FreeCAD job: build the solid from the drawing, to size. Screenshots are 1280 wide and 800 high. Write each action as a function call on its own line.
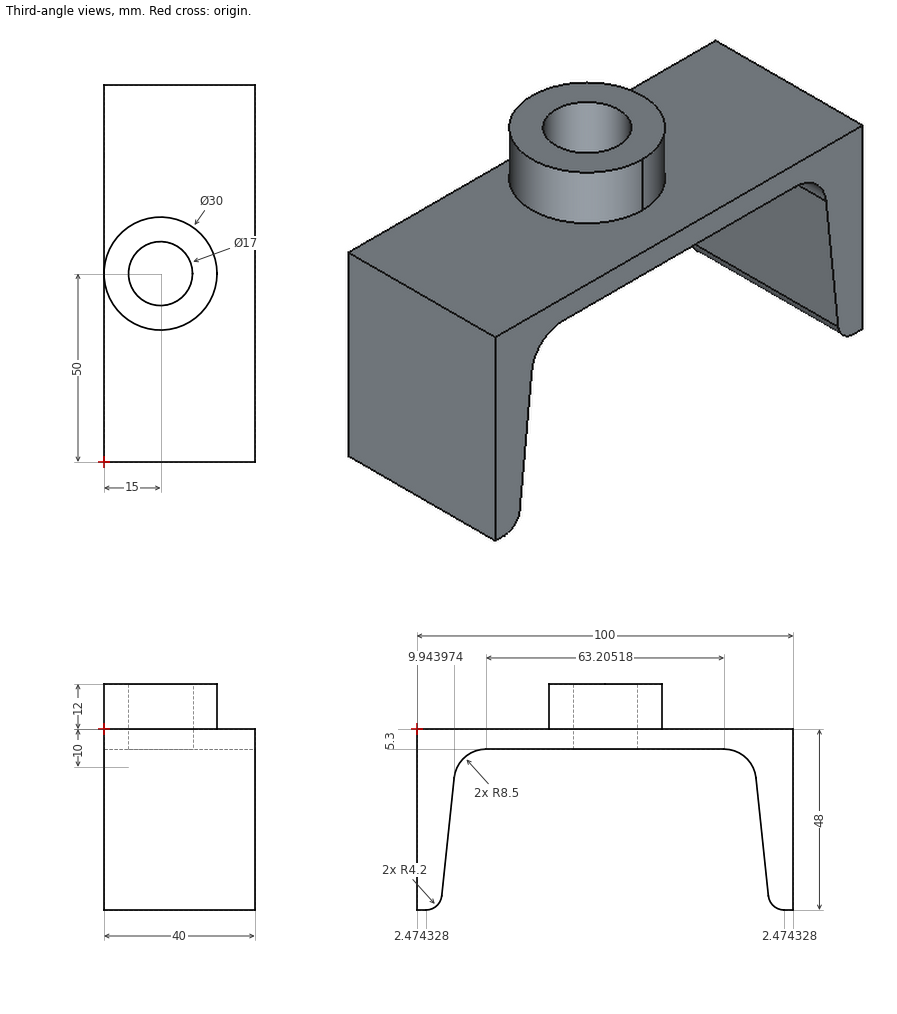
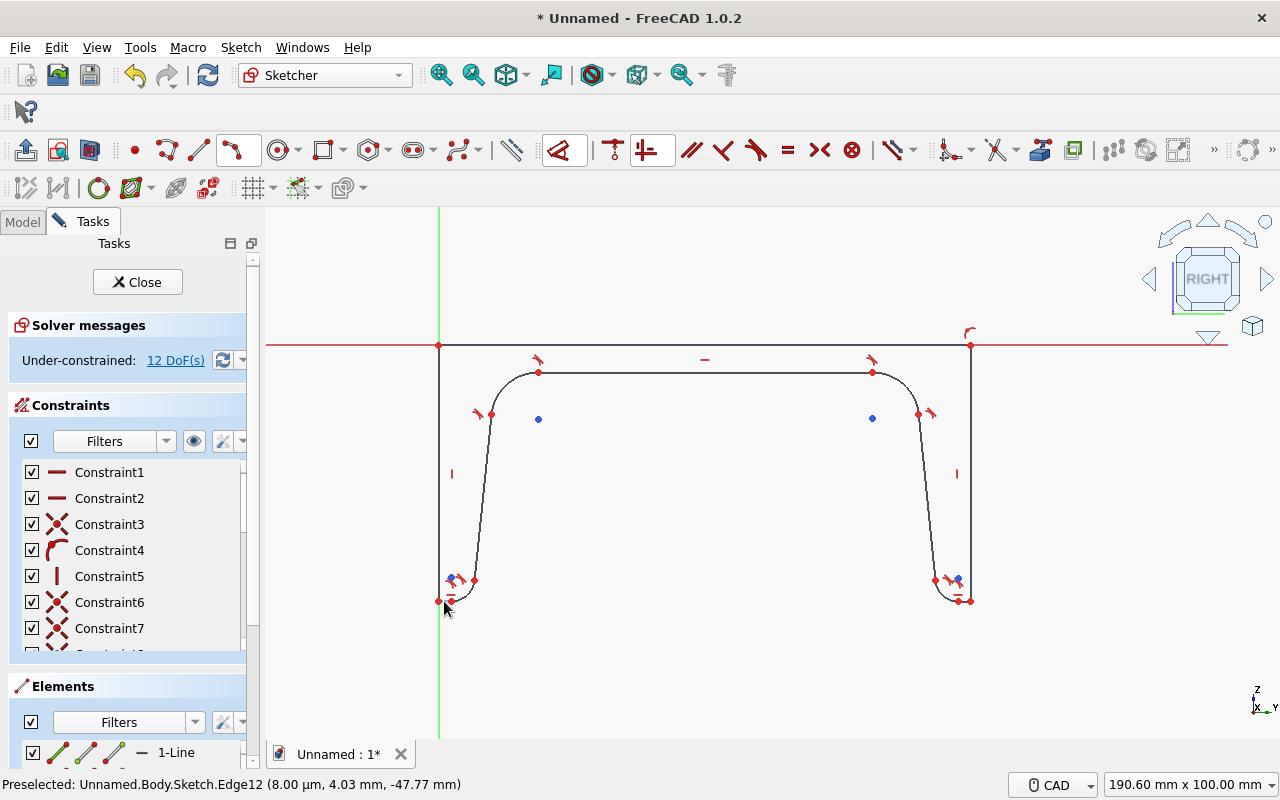
click(518, 377)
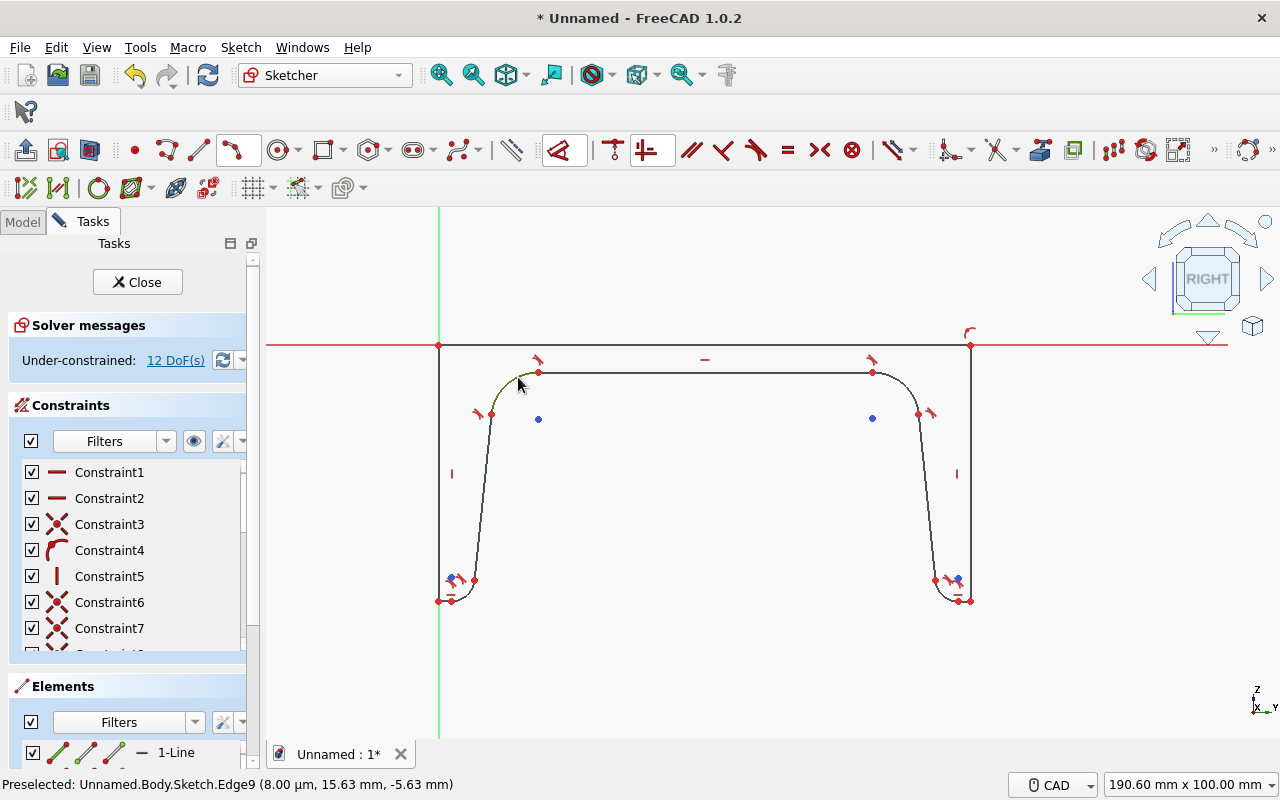
click(912, 395)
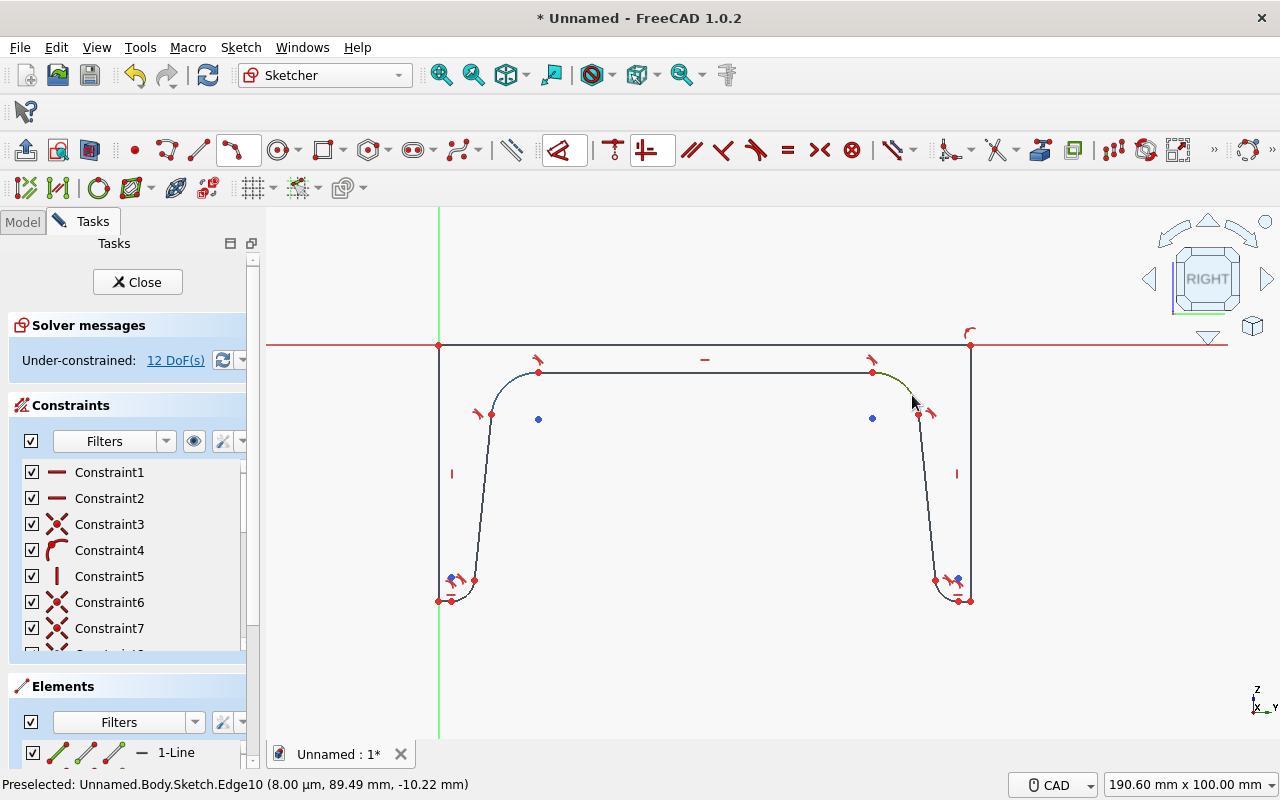
click(788, 150)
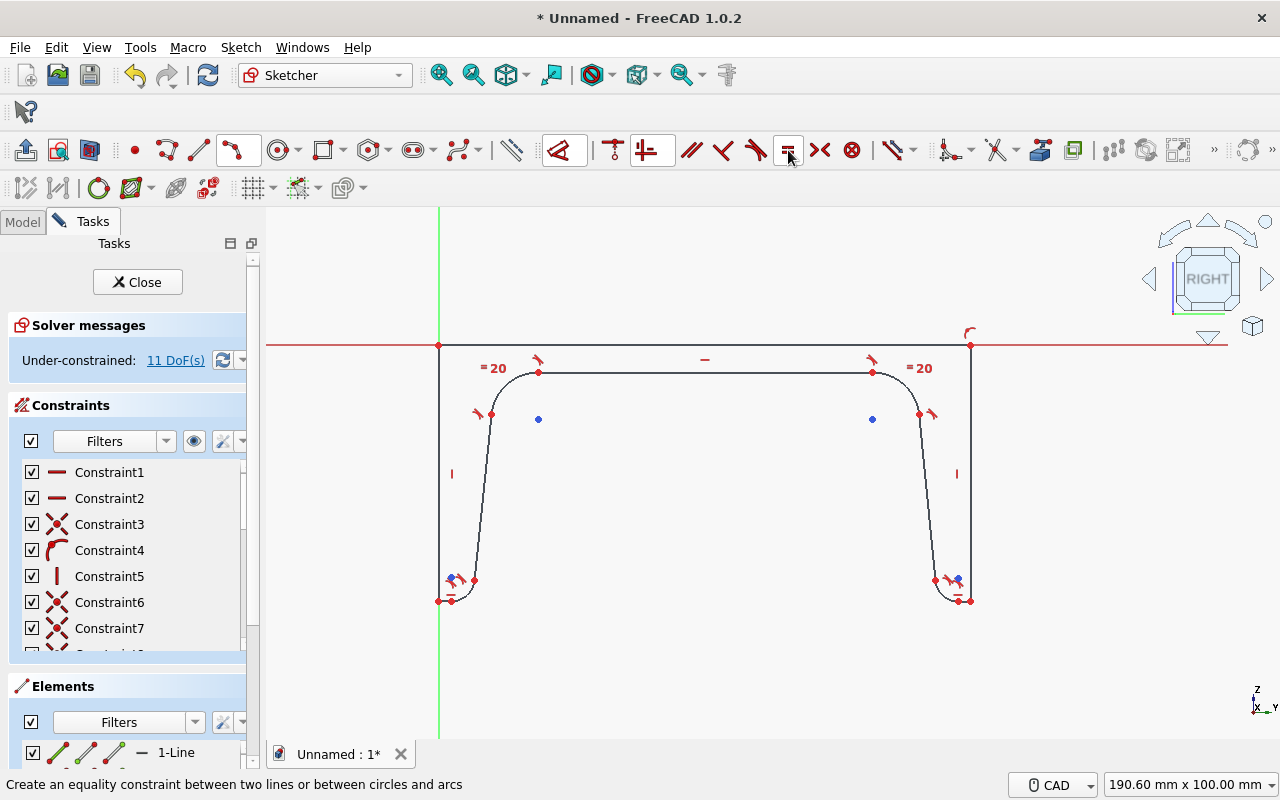
scroll(939, 590, up, 2)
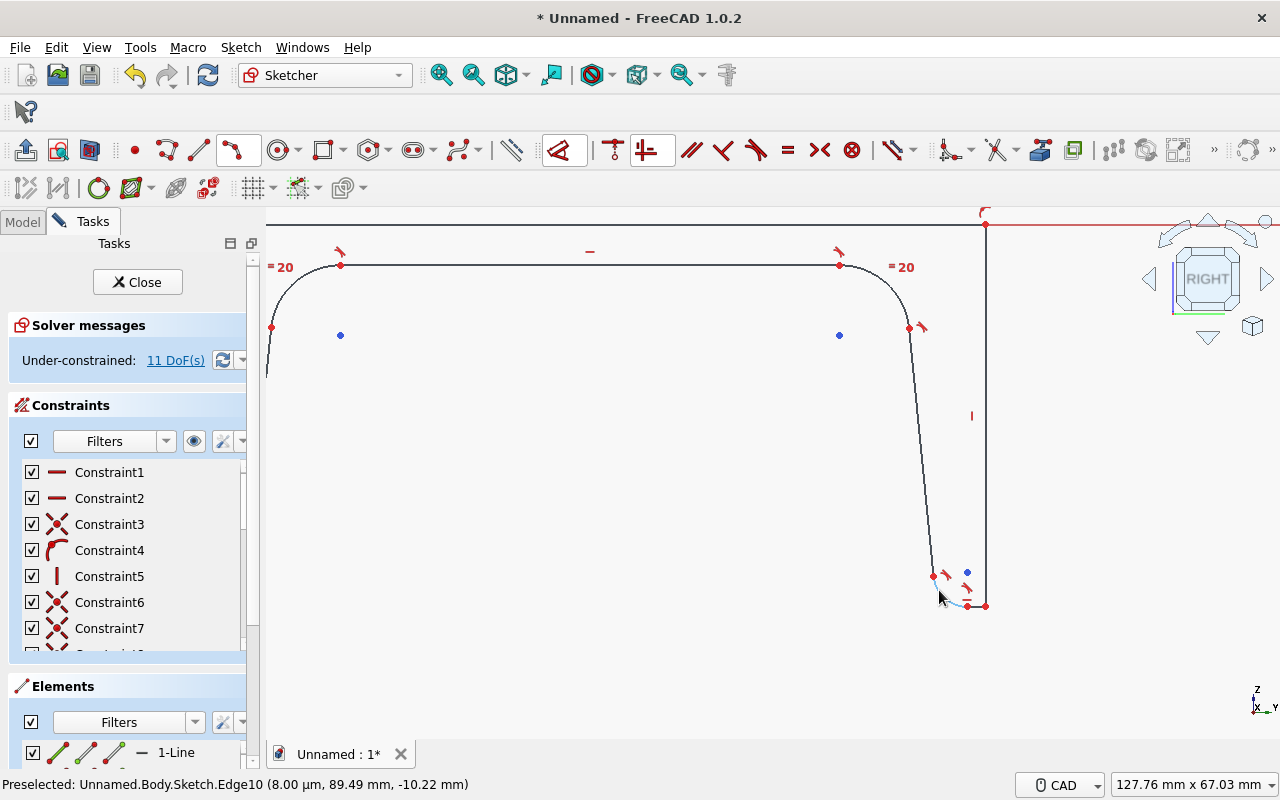
click(938, 590)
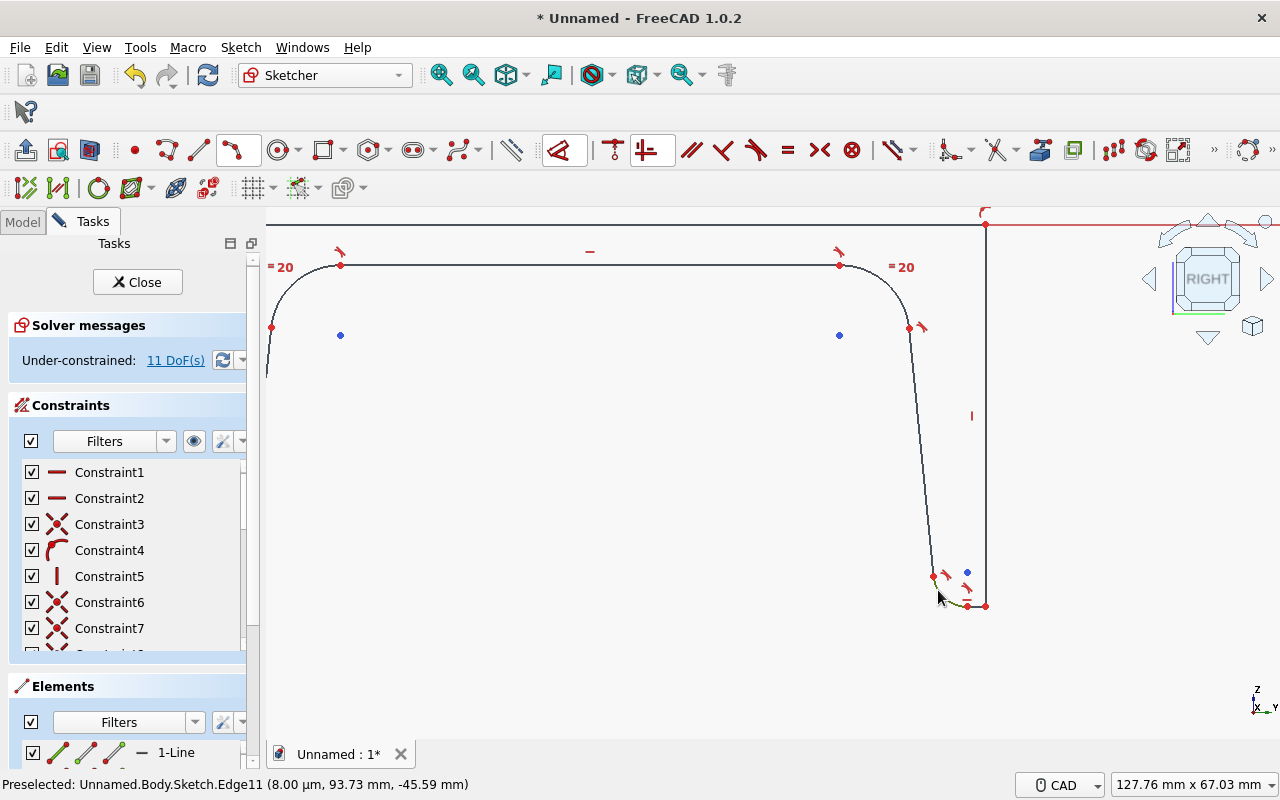
scroll(939, 590, down, 2)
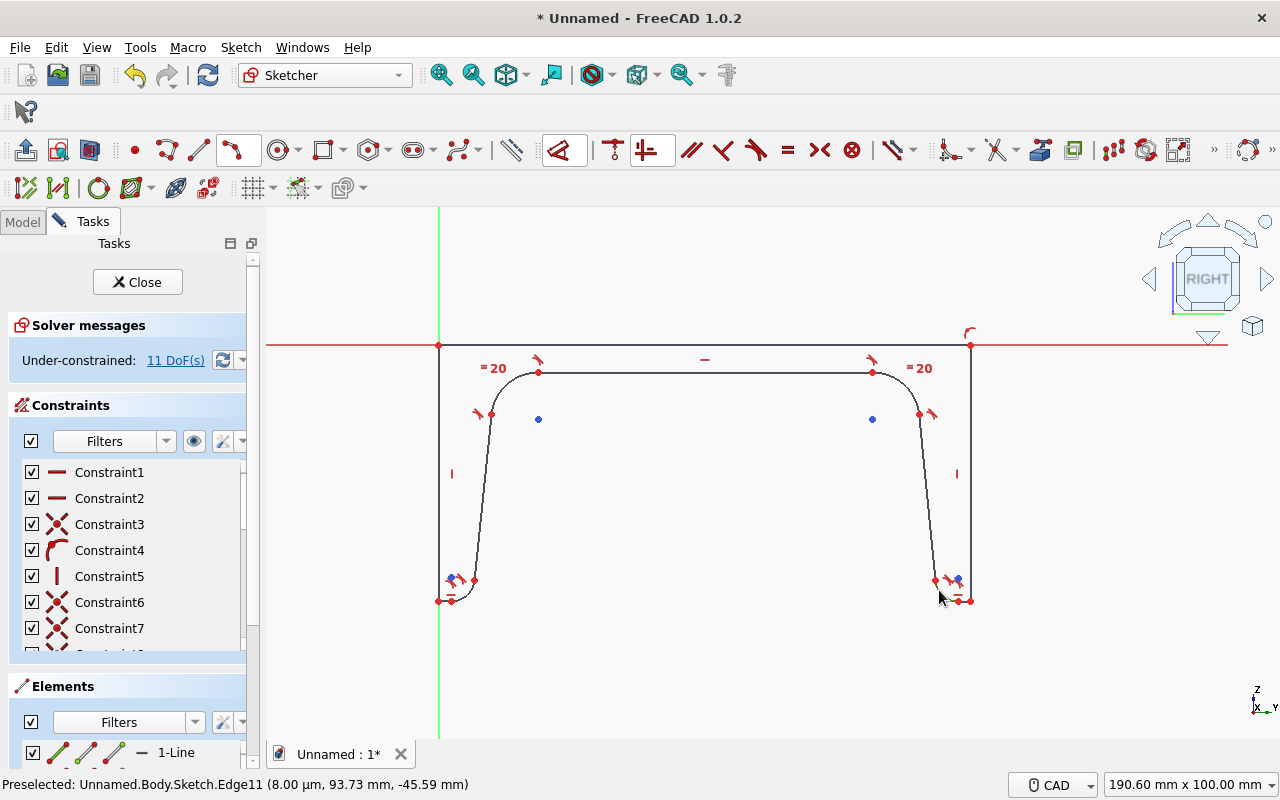
scroll(461, 599, up, 2)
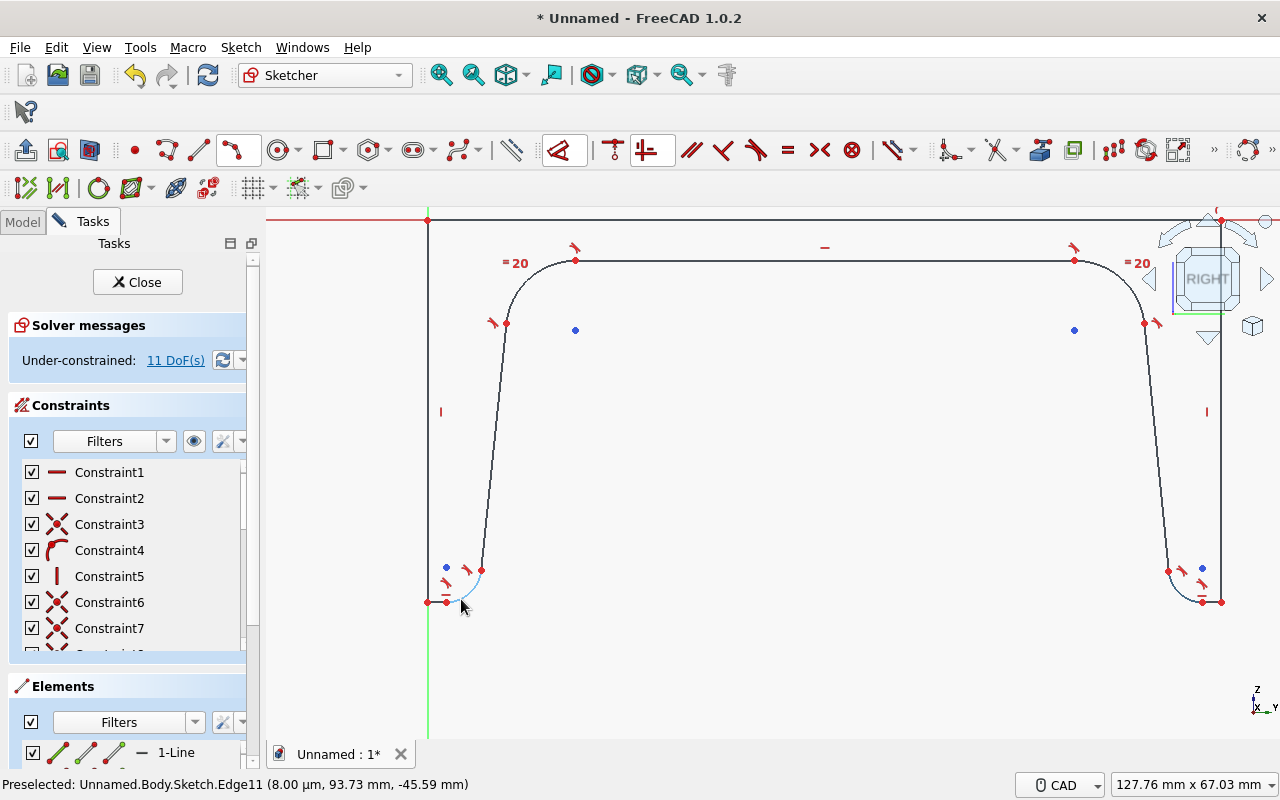
click(461, 599)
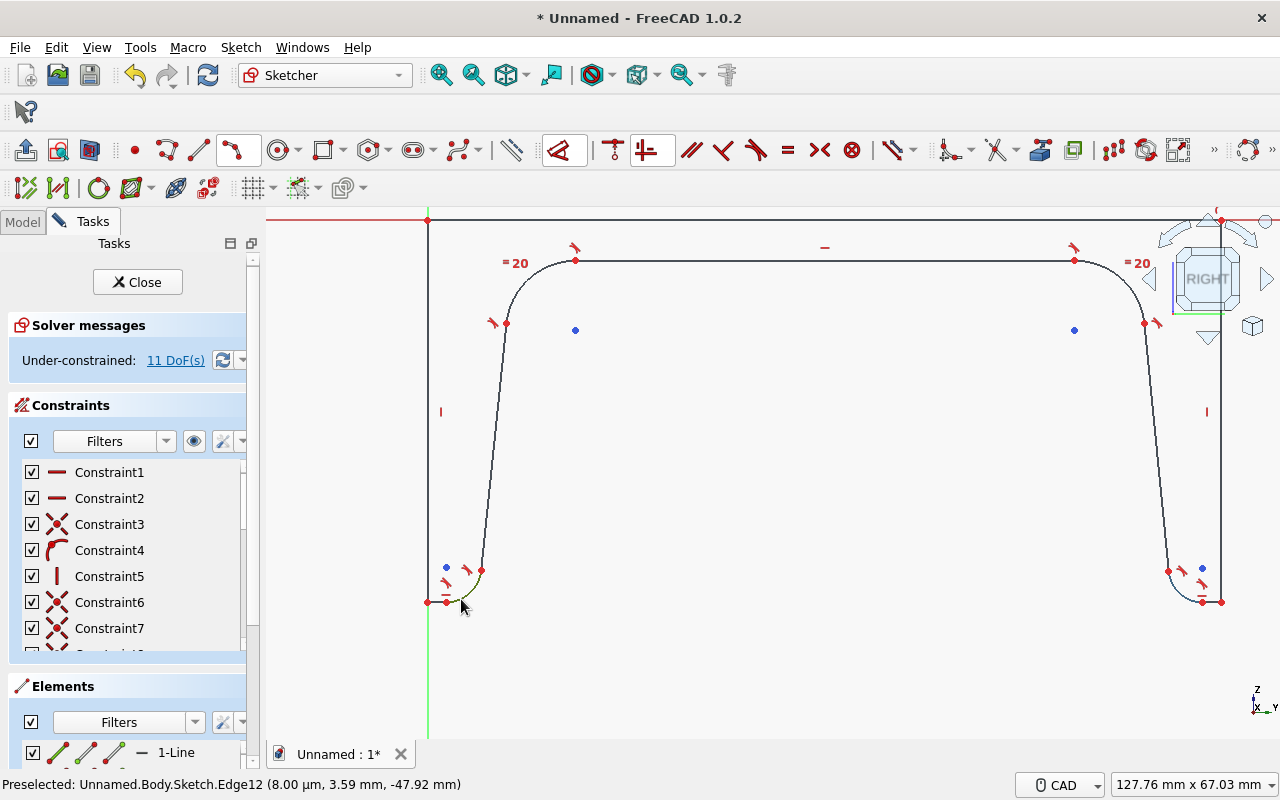
click(788, 150)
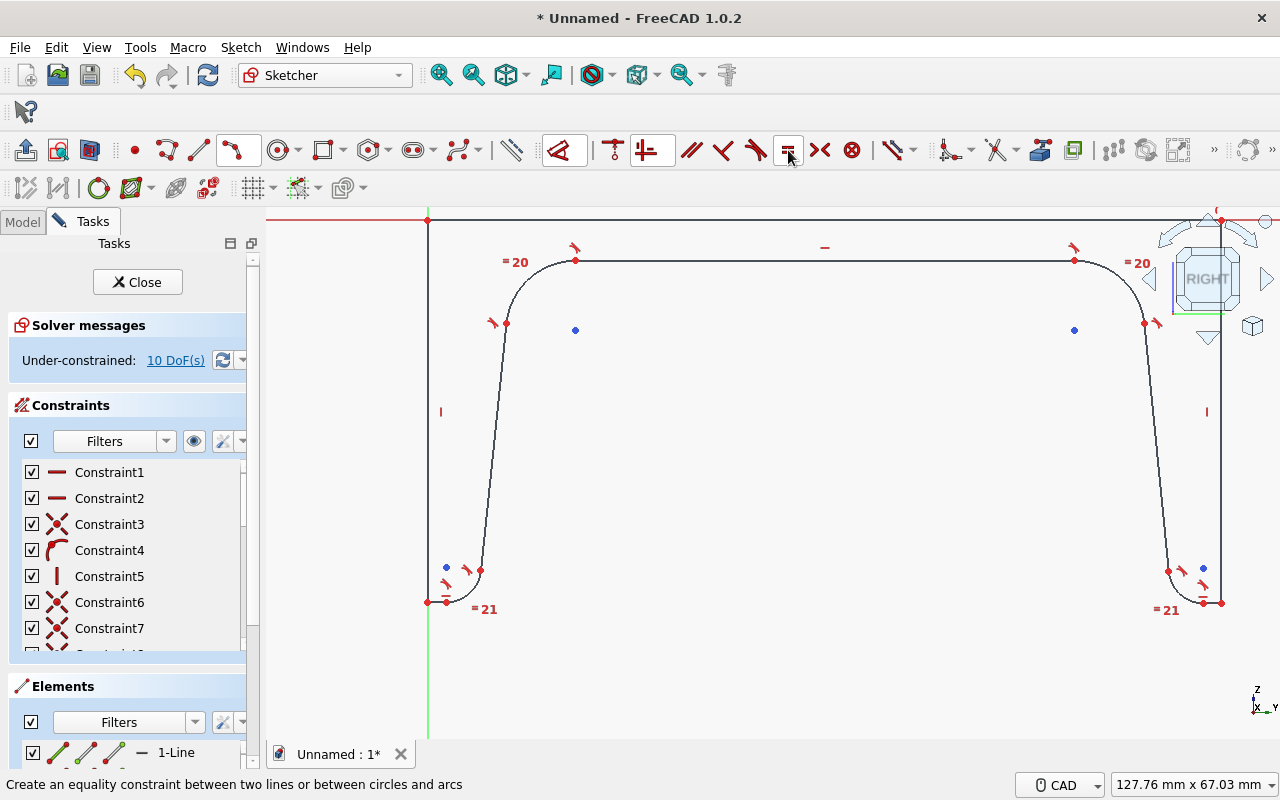
click(558, 150)